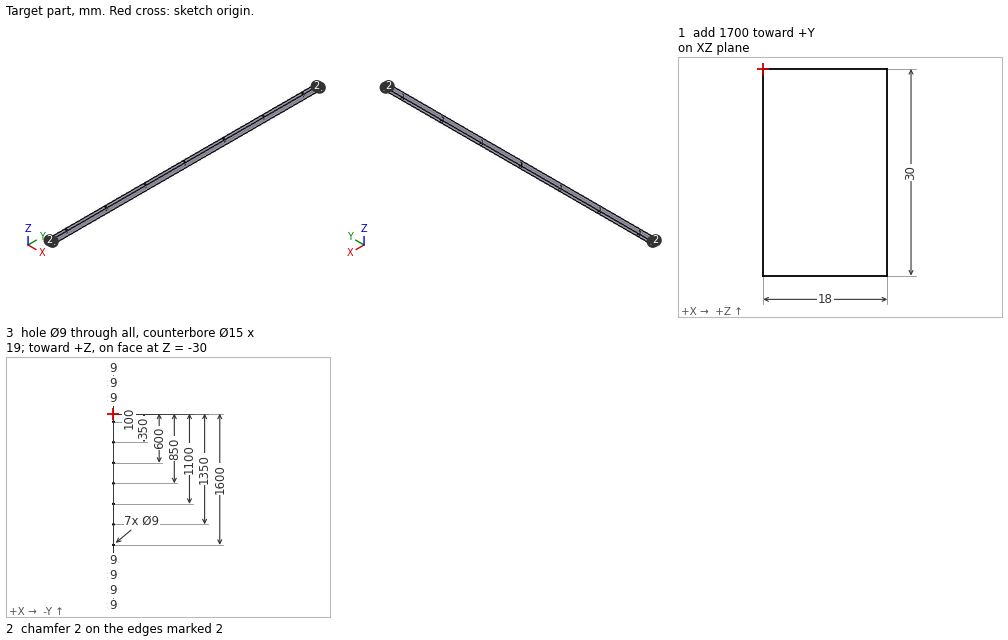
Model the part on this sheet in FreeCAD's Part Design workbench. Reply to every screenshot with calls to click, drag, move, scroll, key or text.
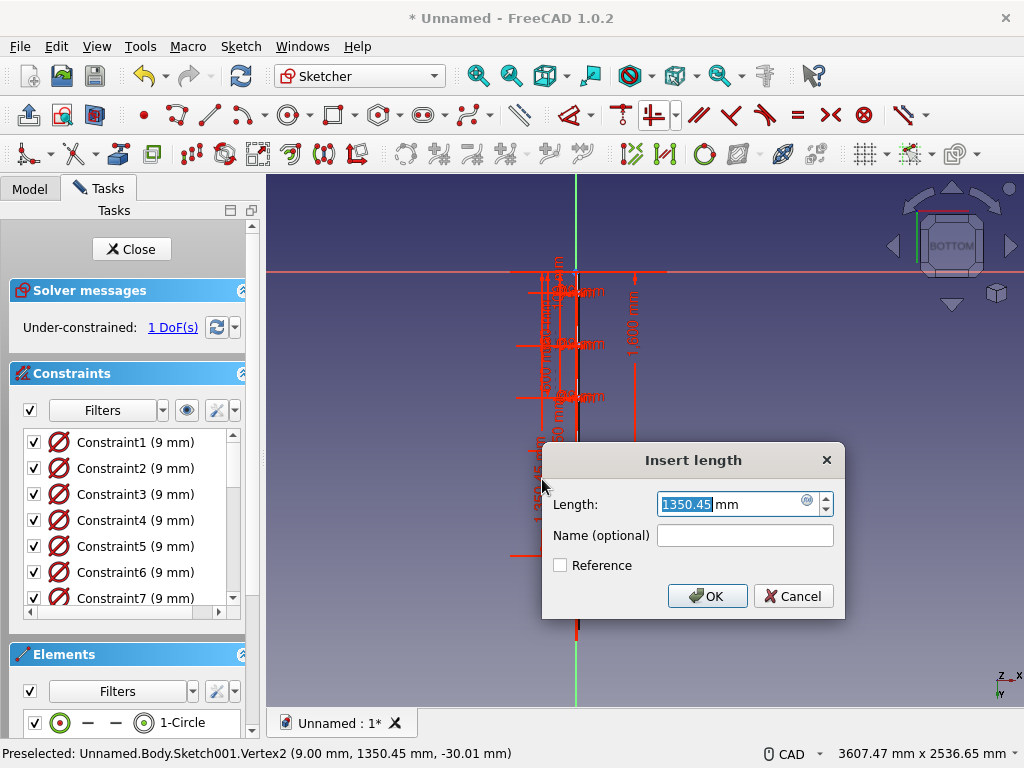
text(1350)
key(Return)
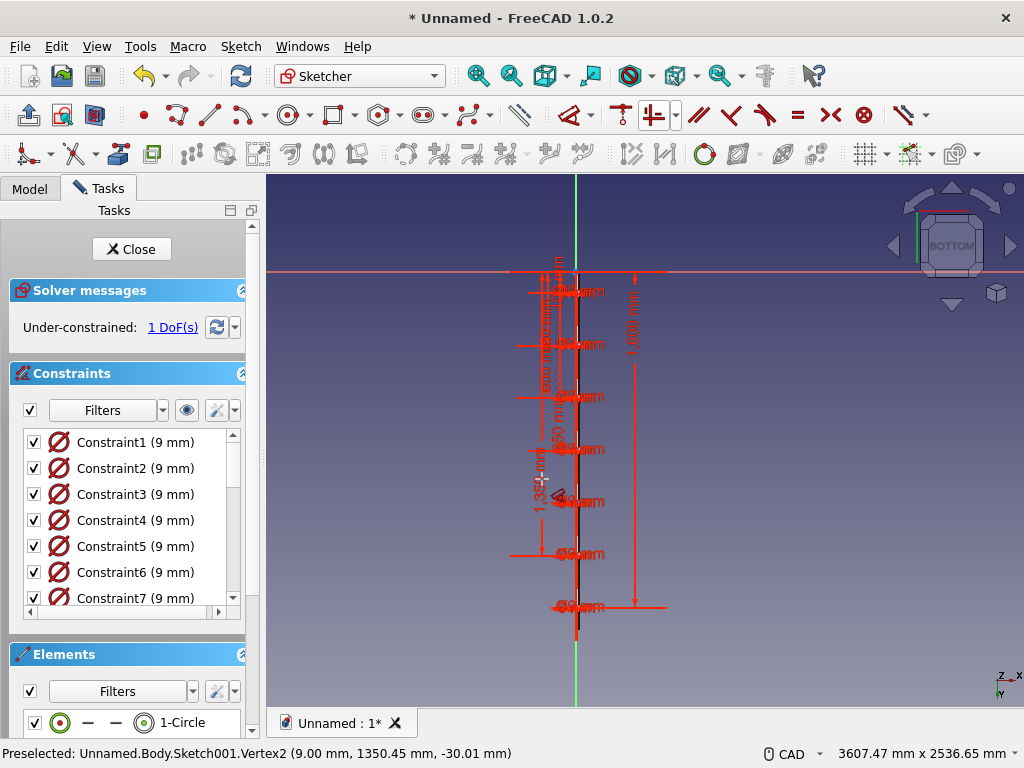
click(577, 503)
click(494, 388)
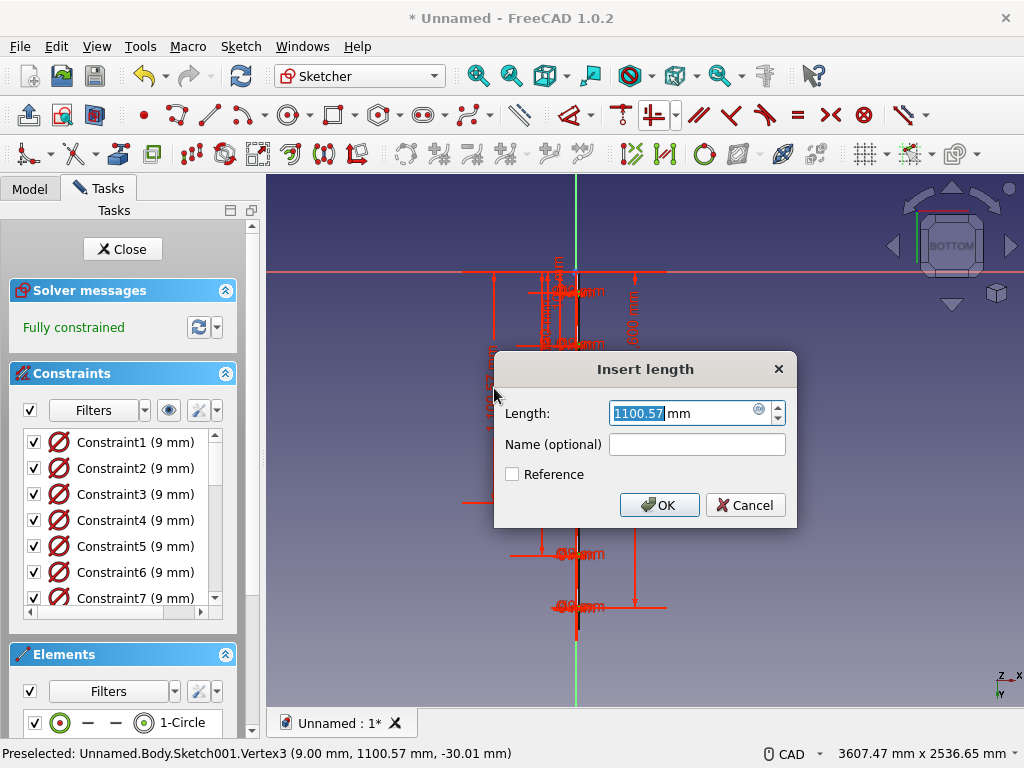
text(1100)
key(Return)
key(Escape)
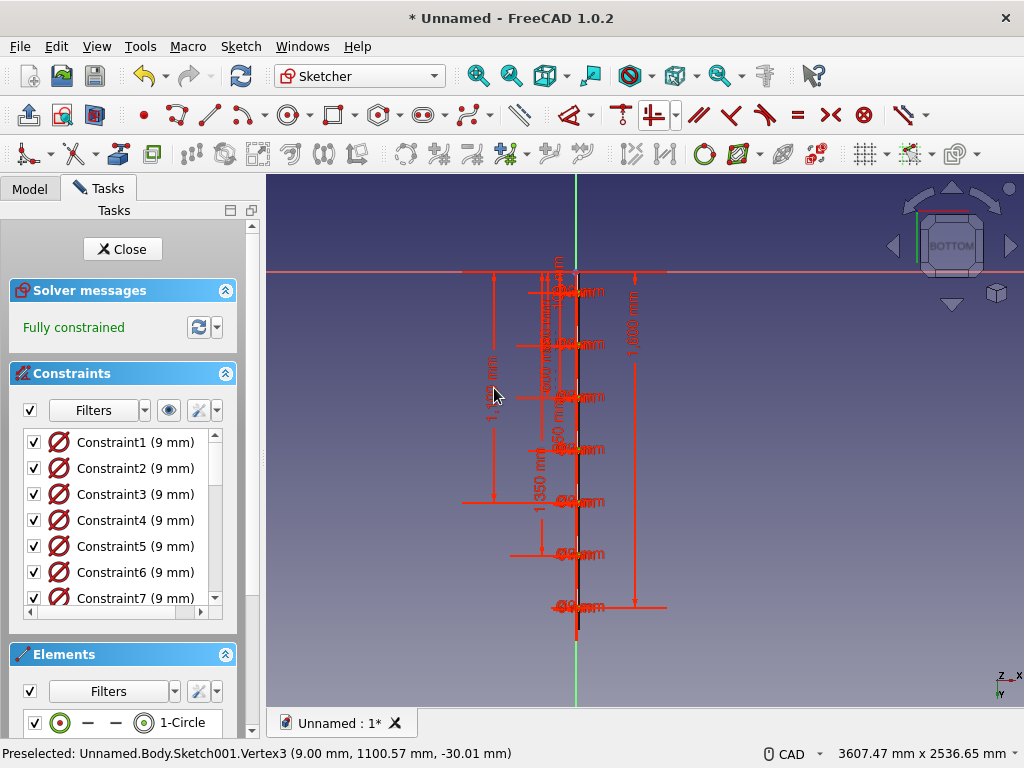
click(123, 249)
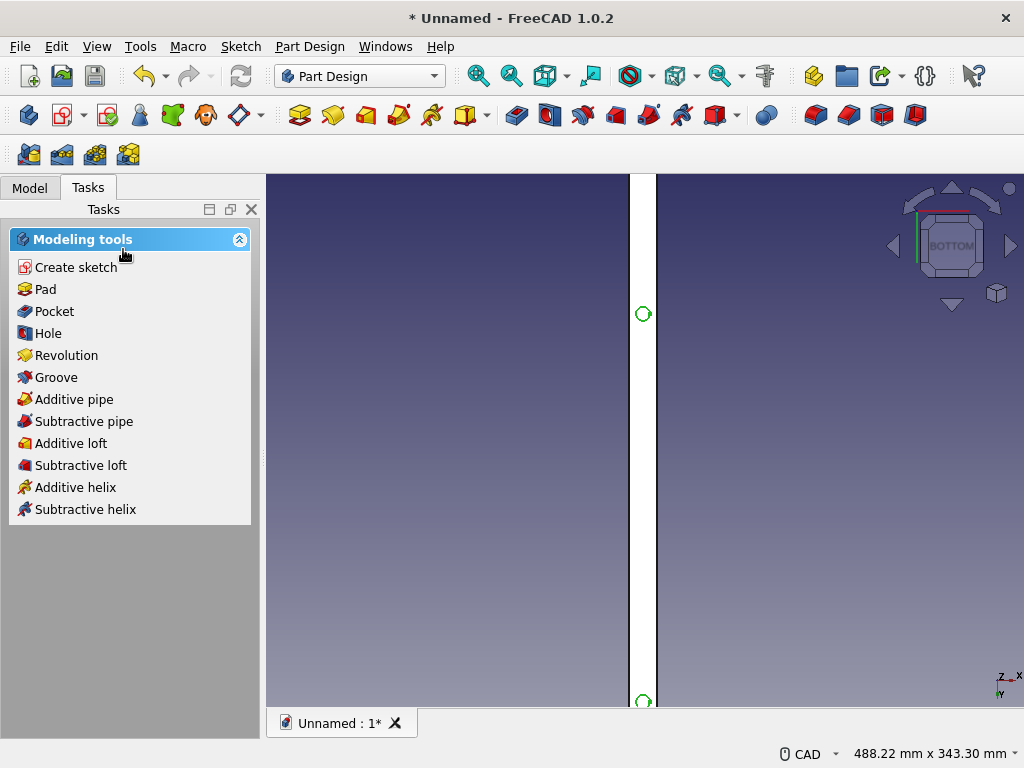
click(550, 116)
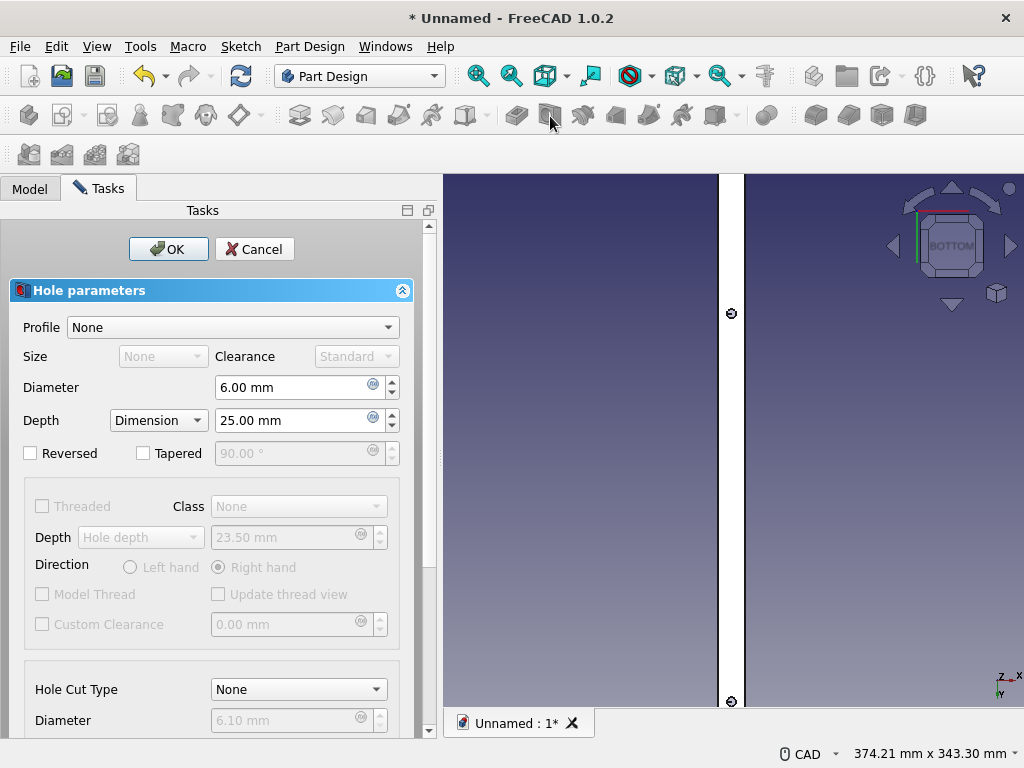
triple_click(300, 388)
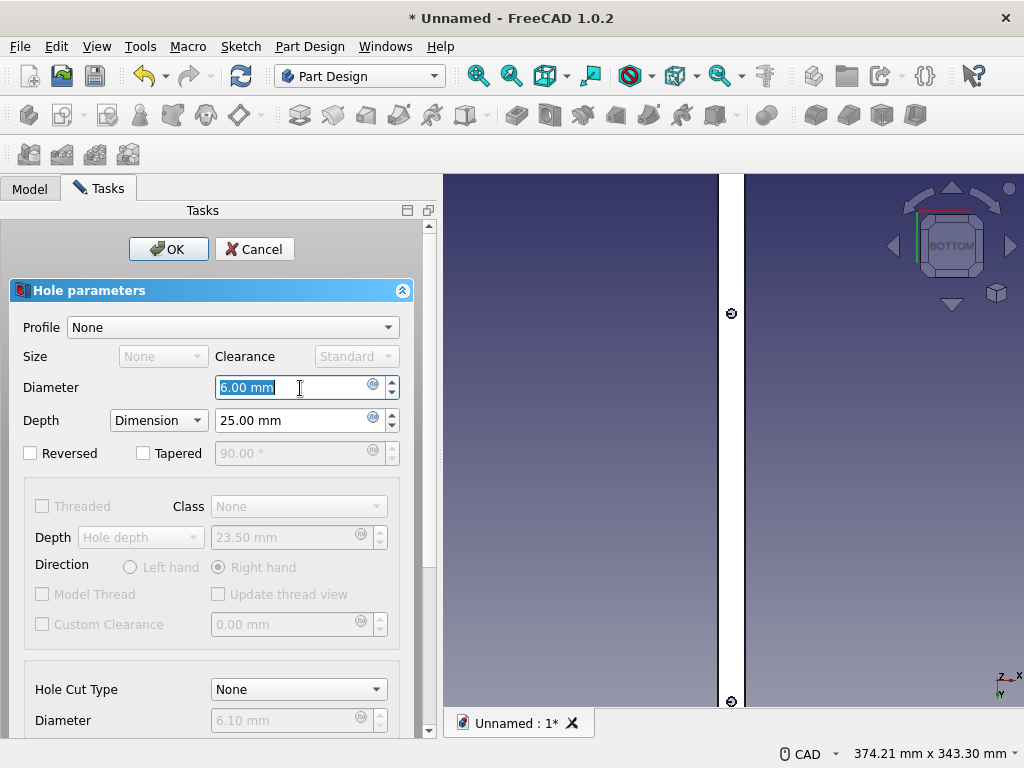
text(9)
key(Tab)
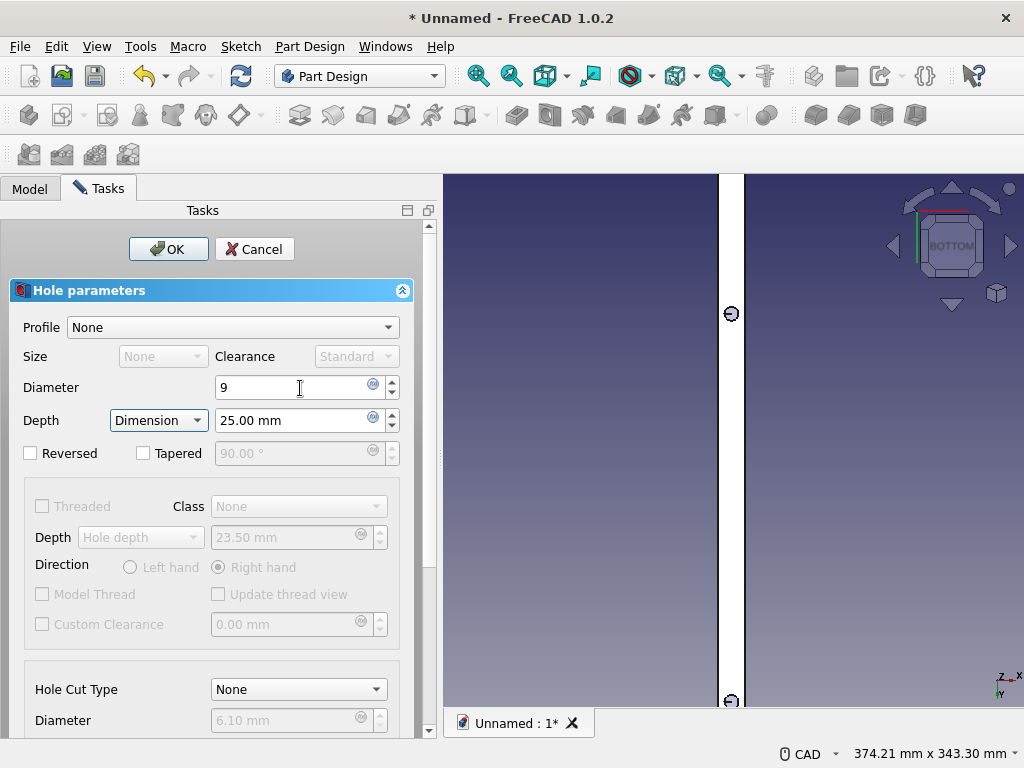
click(160, 420)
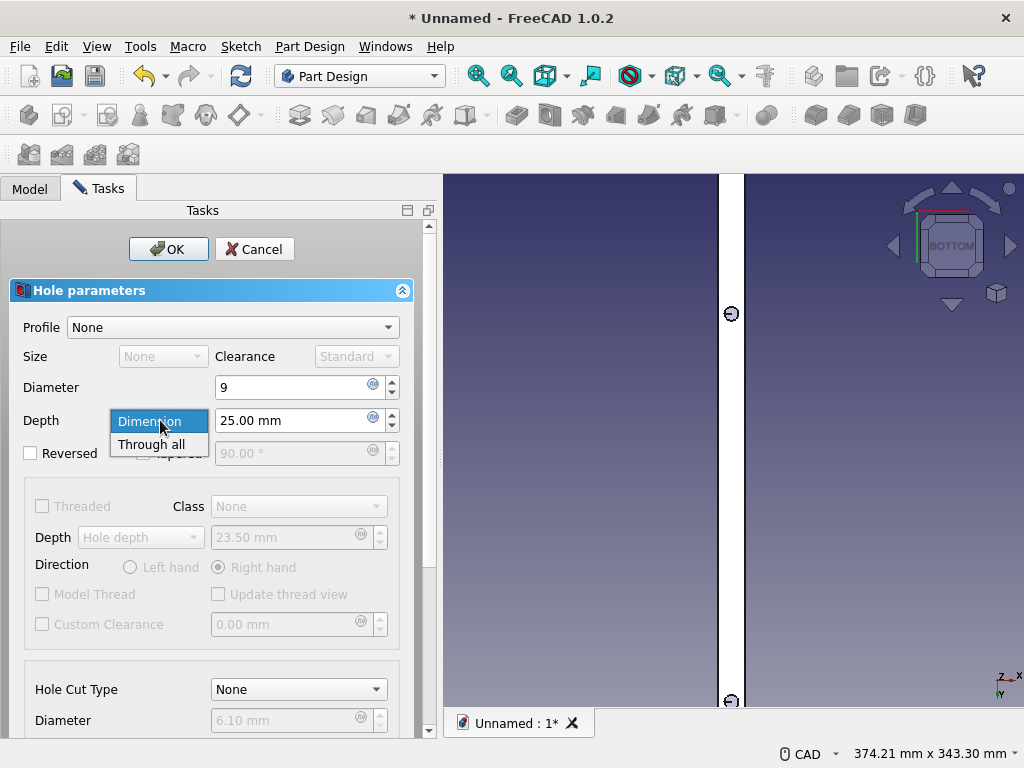
click(158, 444)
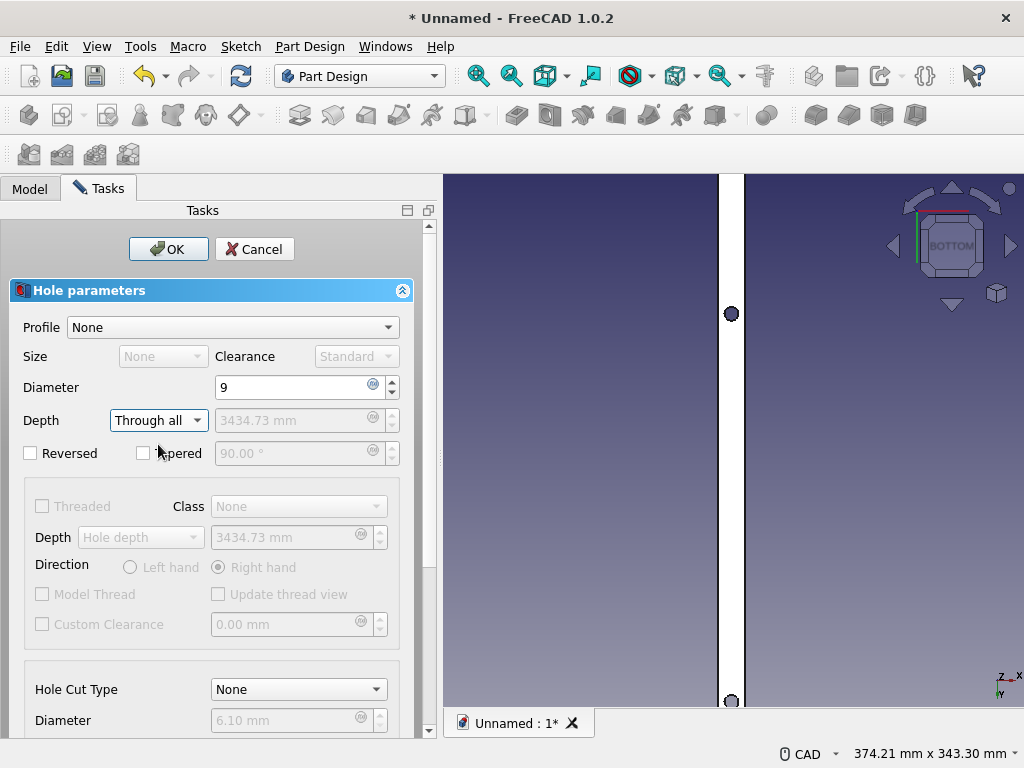
click(300, 690)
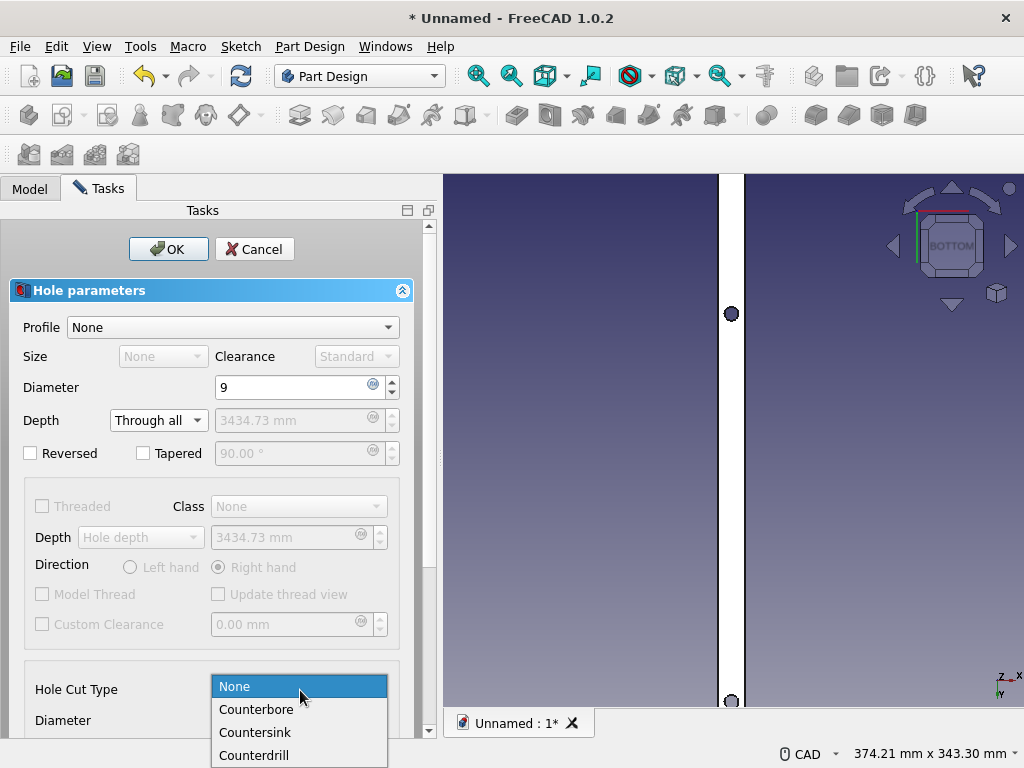
click(298, 710)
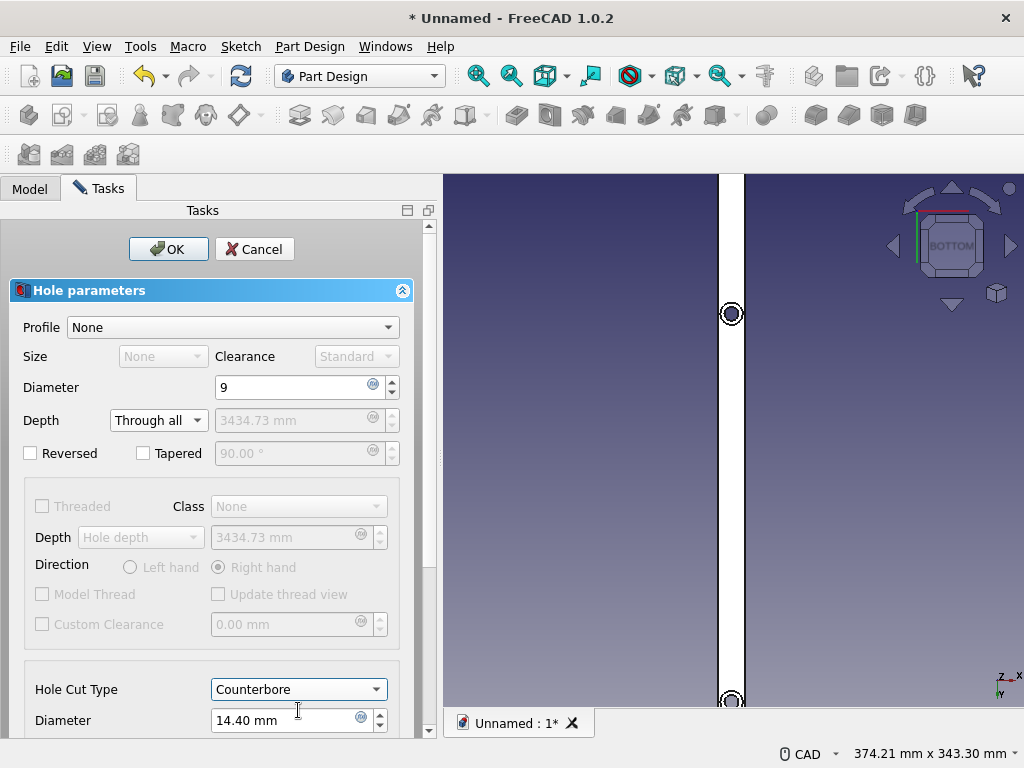
triple_click(292, 720)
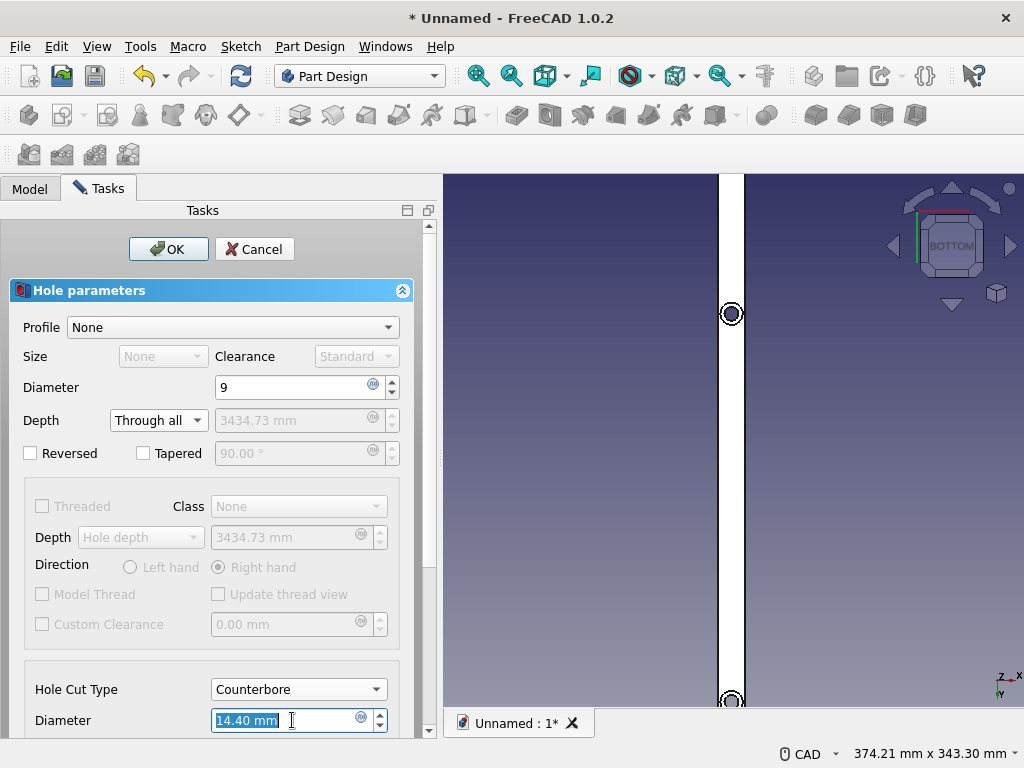
text(15)
key(Tab)